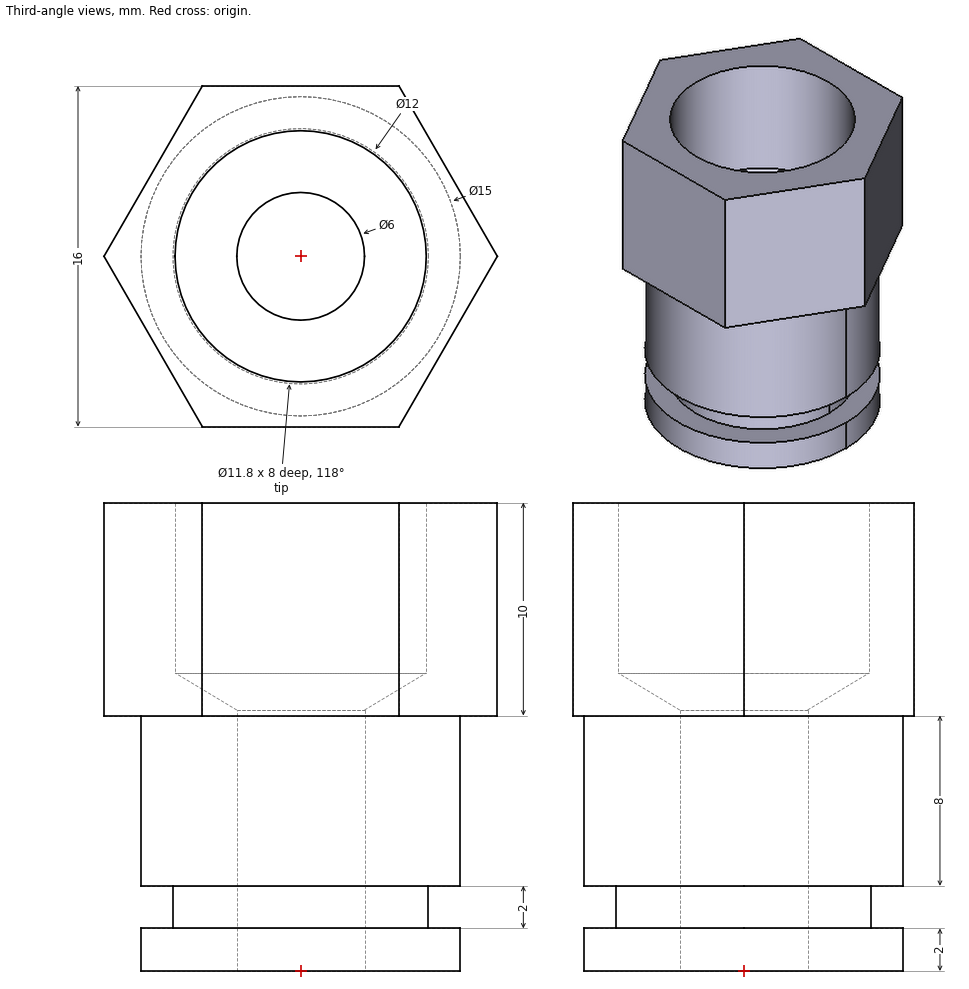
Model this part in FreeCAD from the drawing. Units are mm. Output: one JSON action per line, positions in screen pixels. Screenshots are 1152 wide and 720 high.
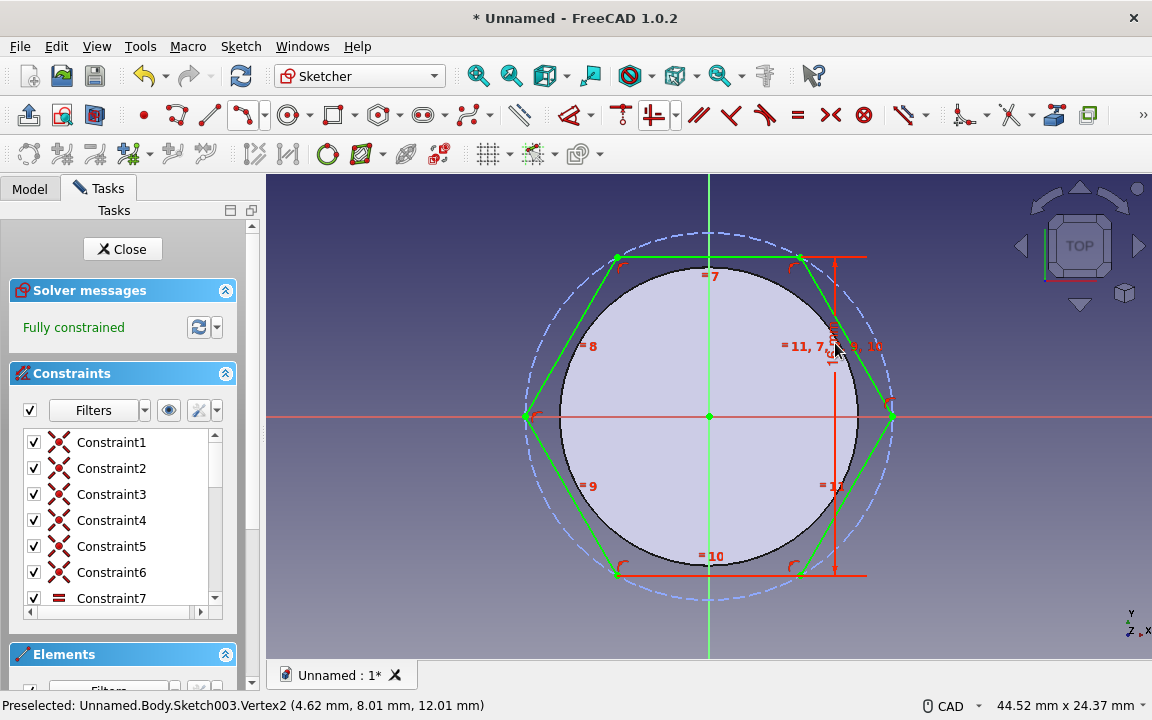
{"action": "left_click", "coordinate": [123, 249]}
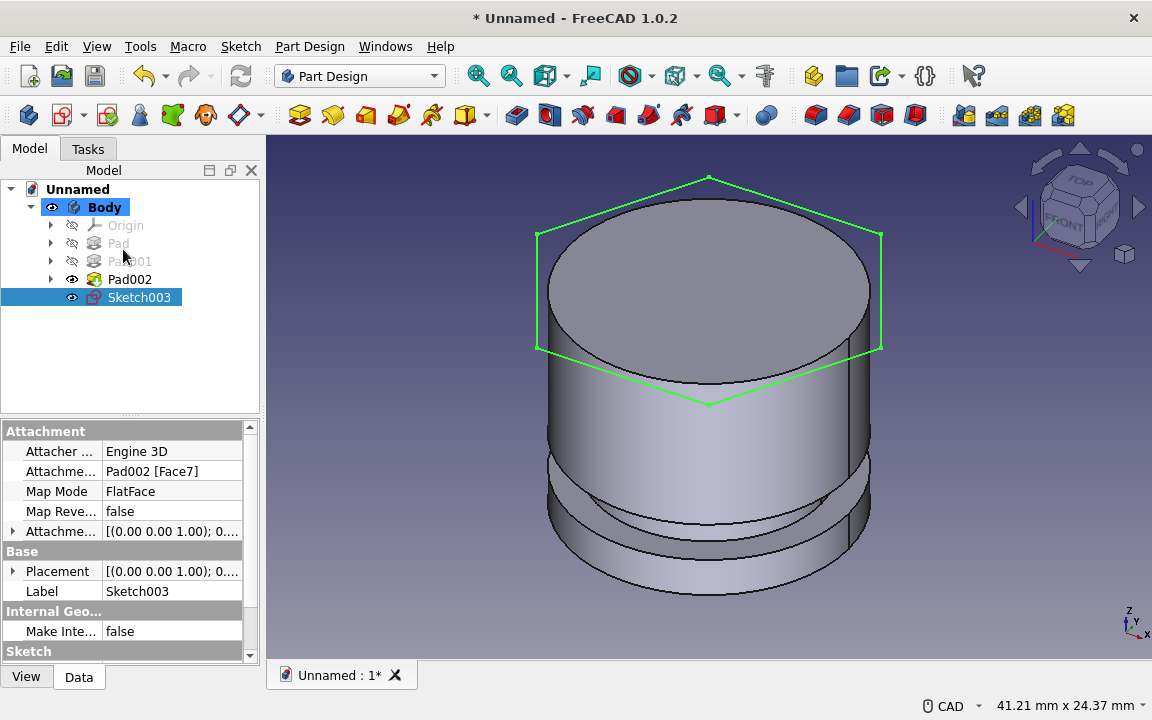
{"action": "left_click", "coordinate": [300, 116]}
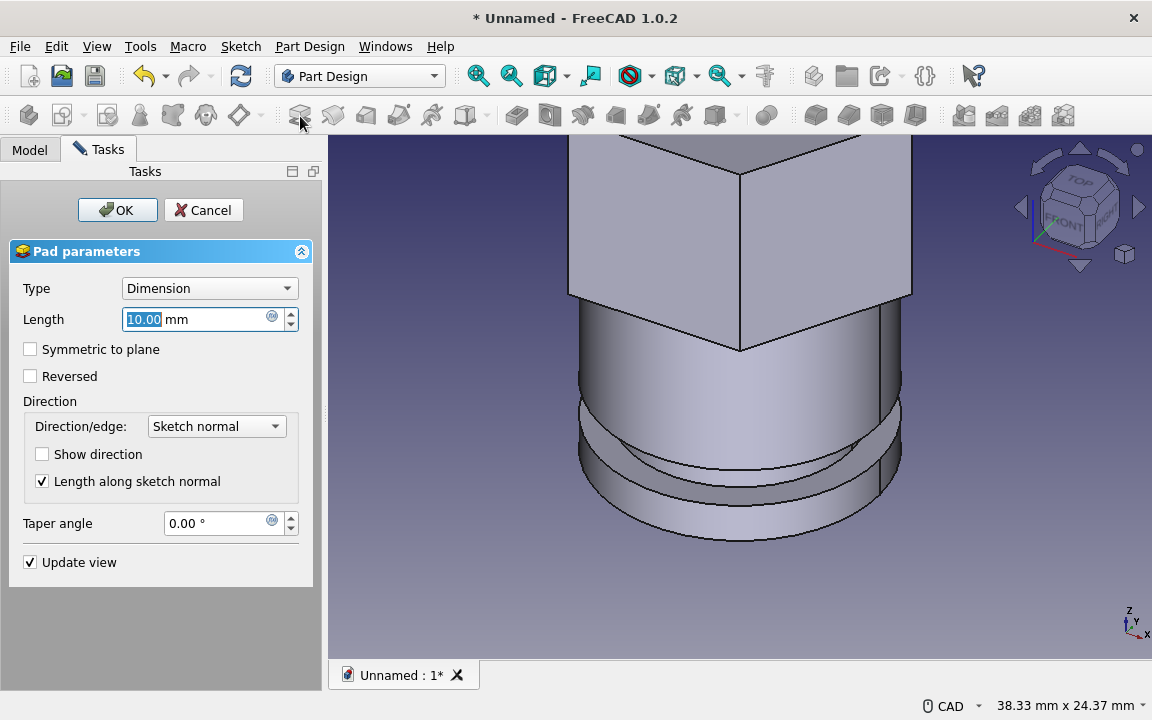
{"action": "type", "text": "10"}
{"action": "key", "text": "Tab"}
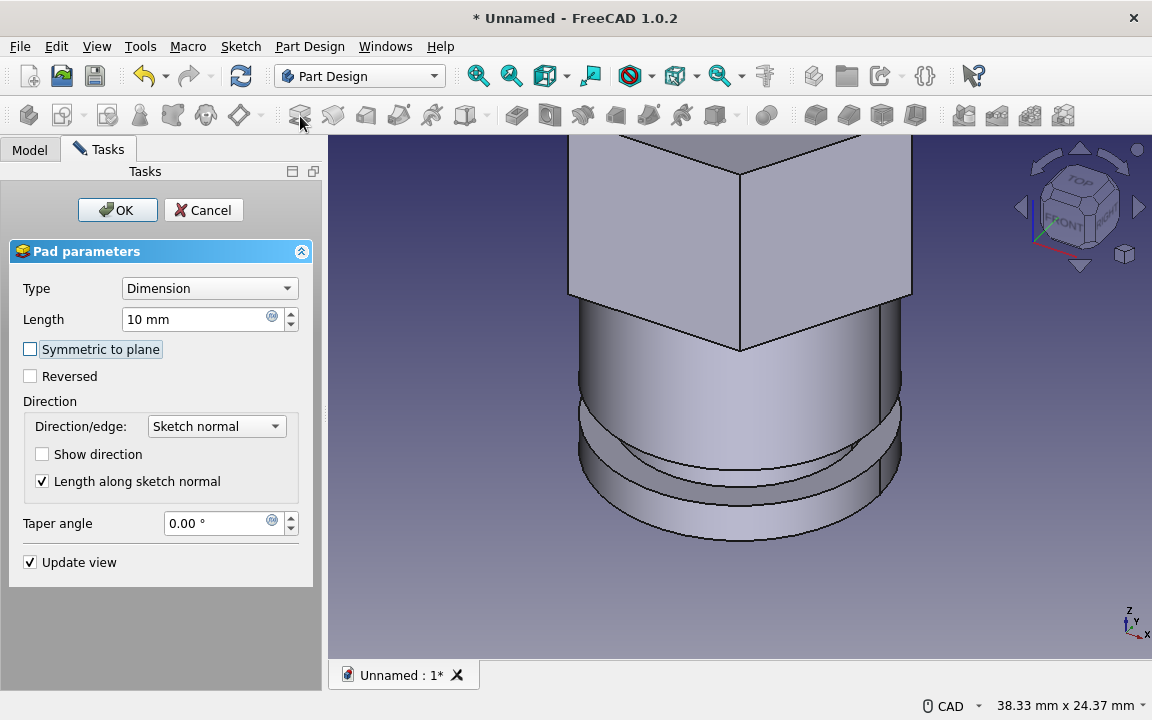
{"action": "left_click", "coordinate": [118, 210]}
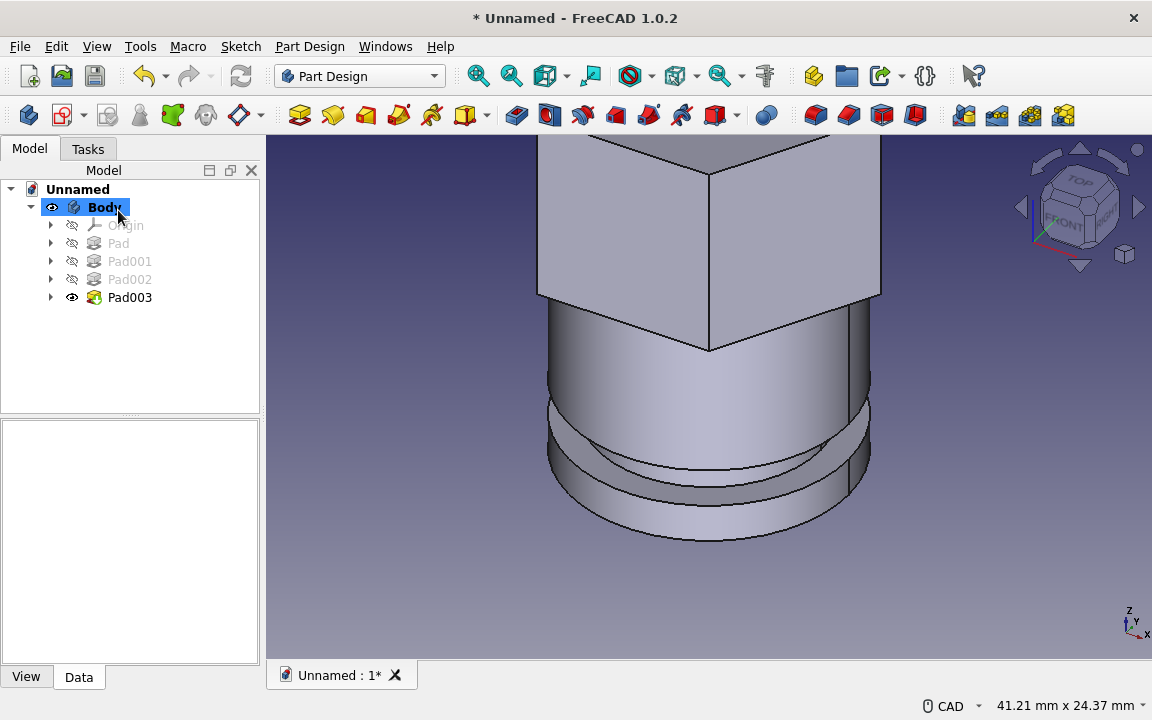
{"action": "key", "text": "v f"}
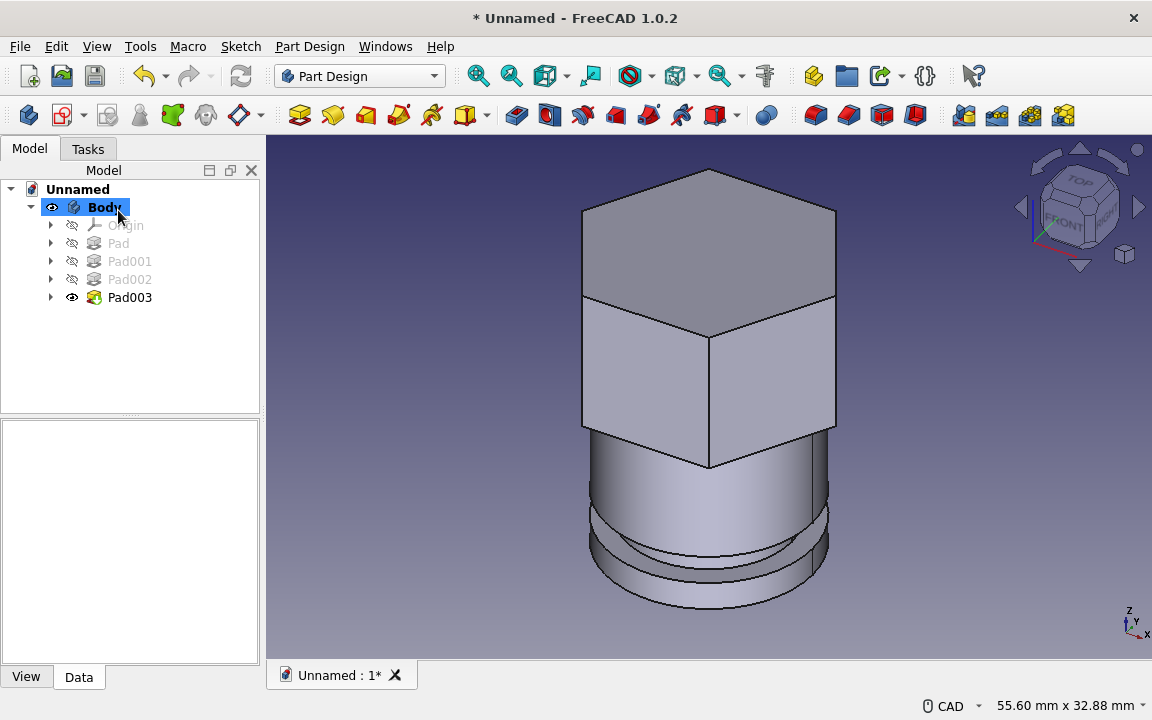
{"action": "left_click", "coordinate": [62, 116]}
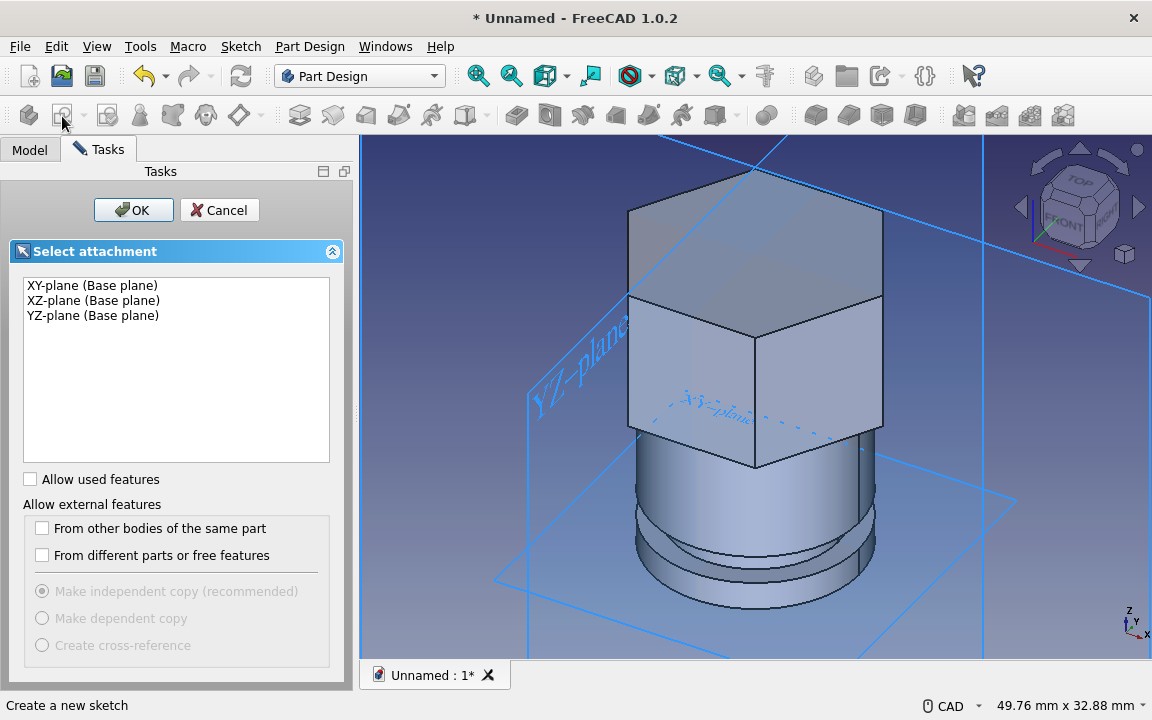
{"action": "left_click", "coordinate": [84, 286]}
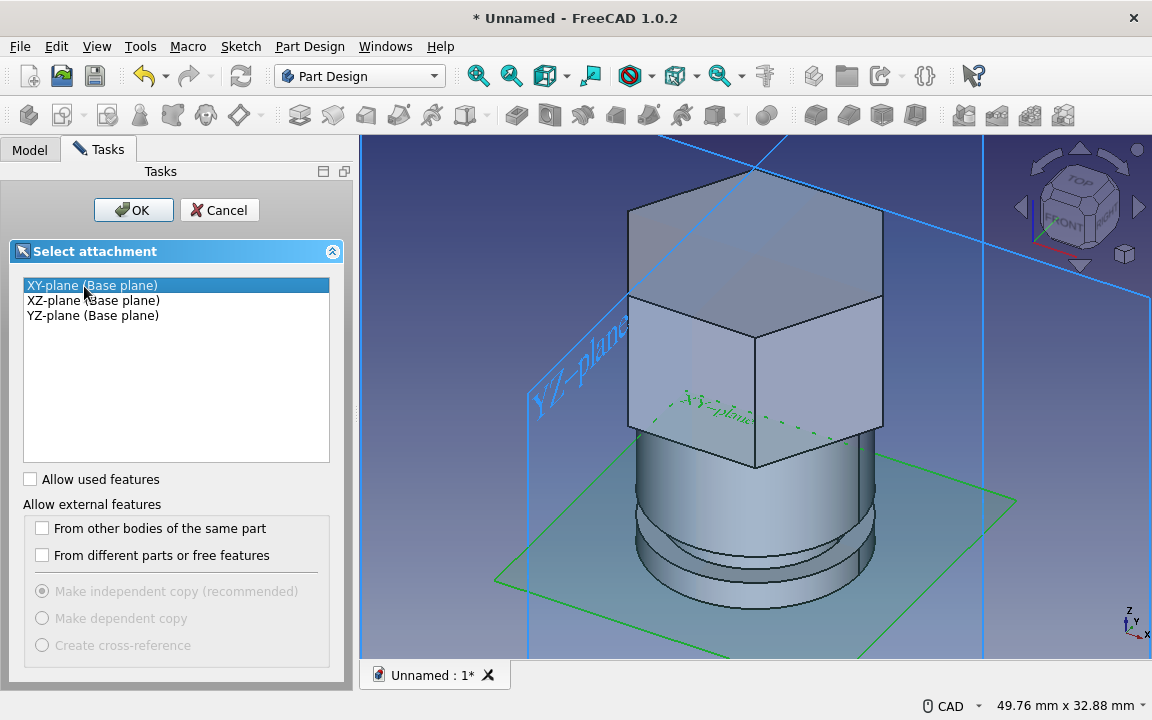
{"action": "left_click", "coordinate": [134, 210]}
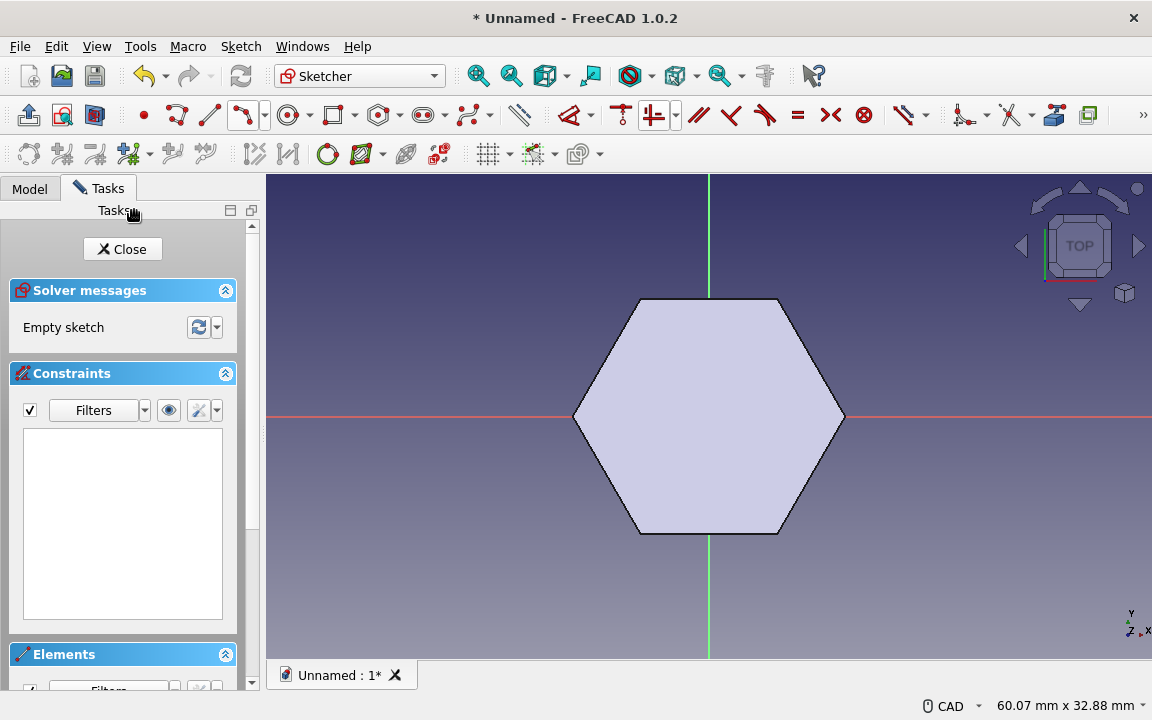
{"action": "key", "text": "q s"}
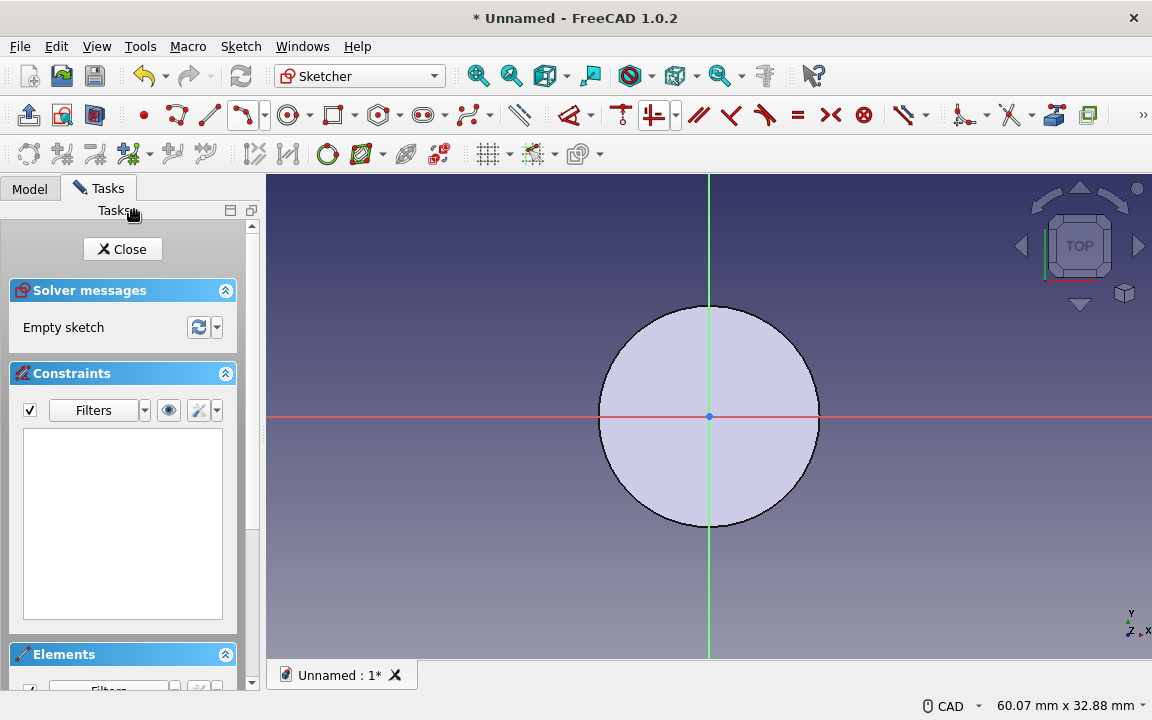
{"action": "scroll", "coordinate": [739, 416], "scroll_direction": "up", "scroll_amount": 6}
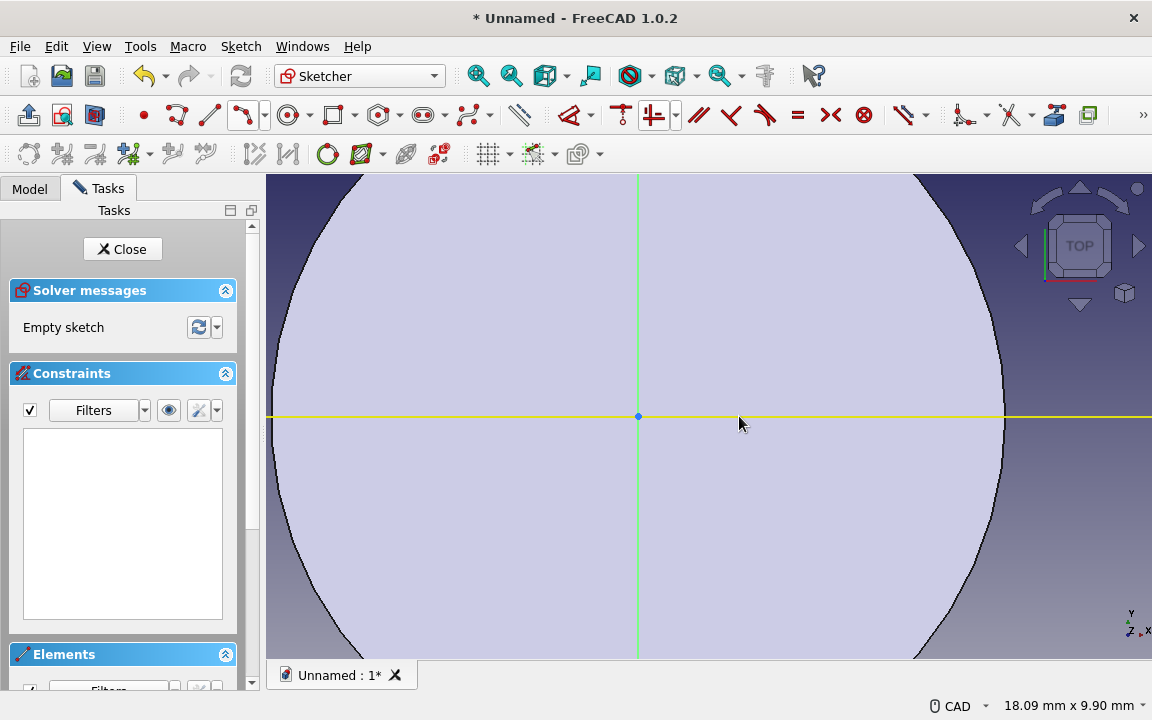
{"action": "key", "text": "g c"}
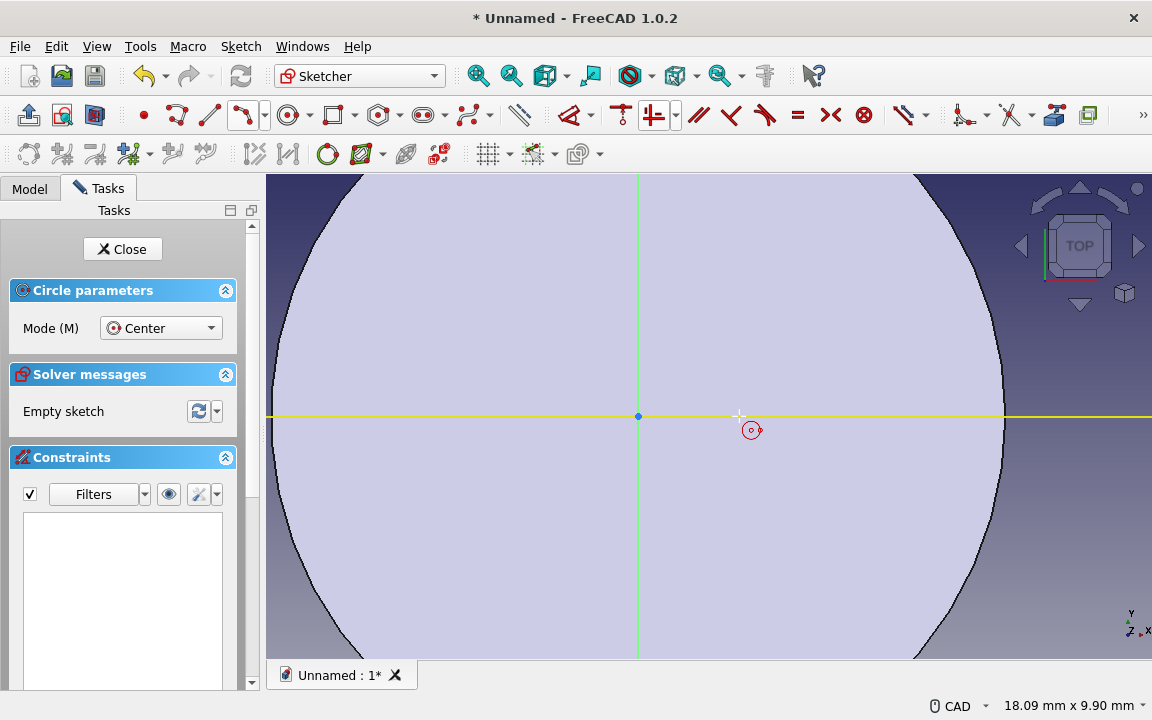
{"action": "left_click", "coordinate": [638, 416]}
{"action": "left_click", "coordinate": [742, 313]}
{"action": "key", "text": "Escape"}